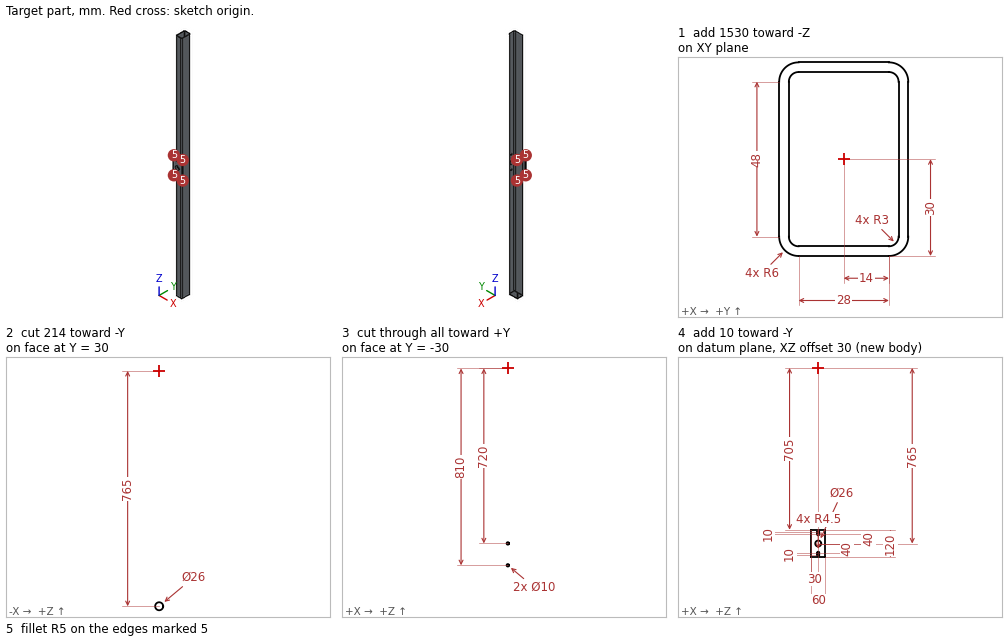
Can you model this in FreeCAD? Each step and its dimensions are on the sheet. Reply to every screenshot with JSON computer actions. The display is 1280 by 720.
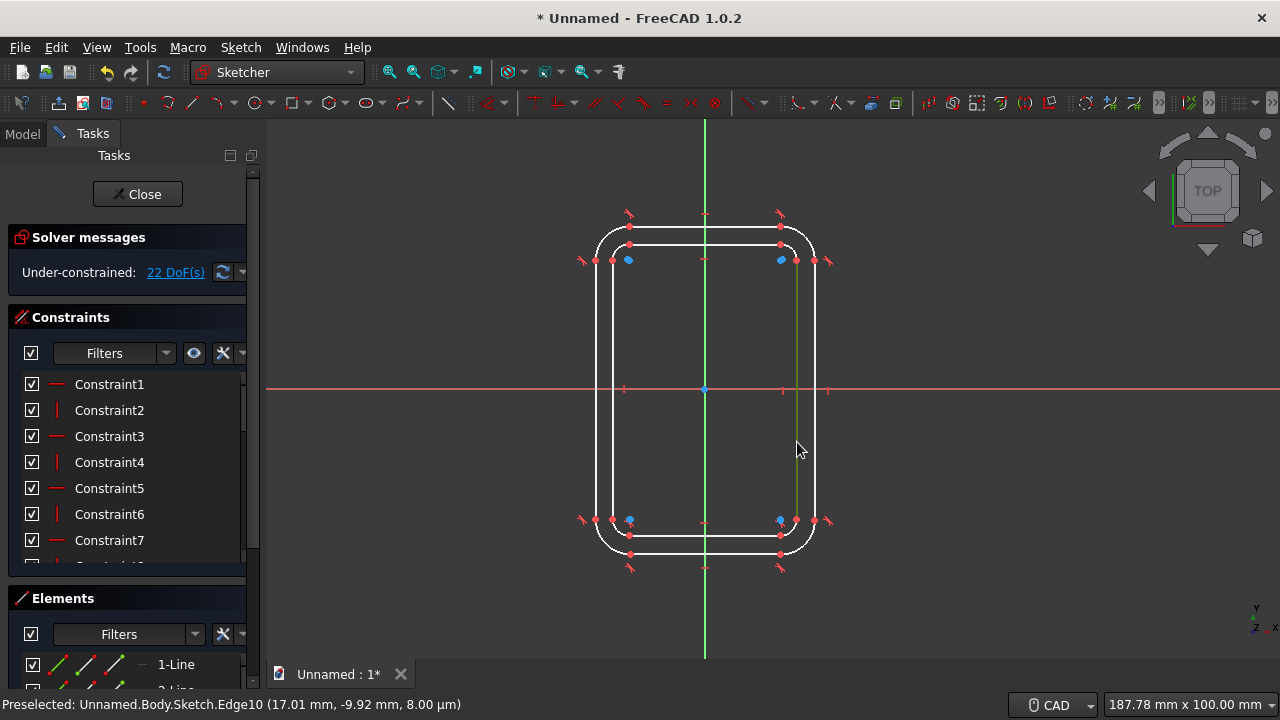
{"action": "left_click", "coordinate": [792, 531]}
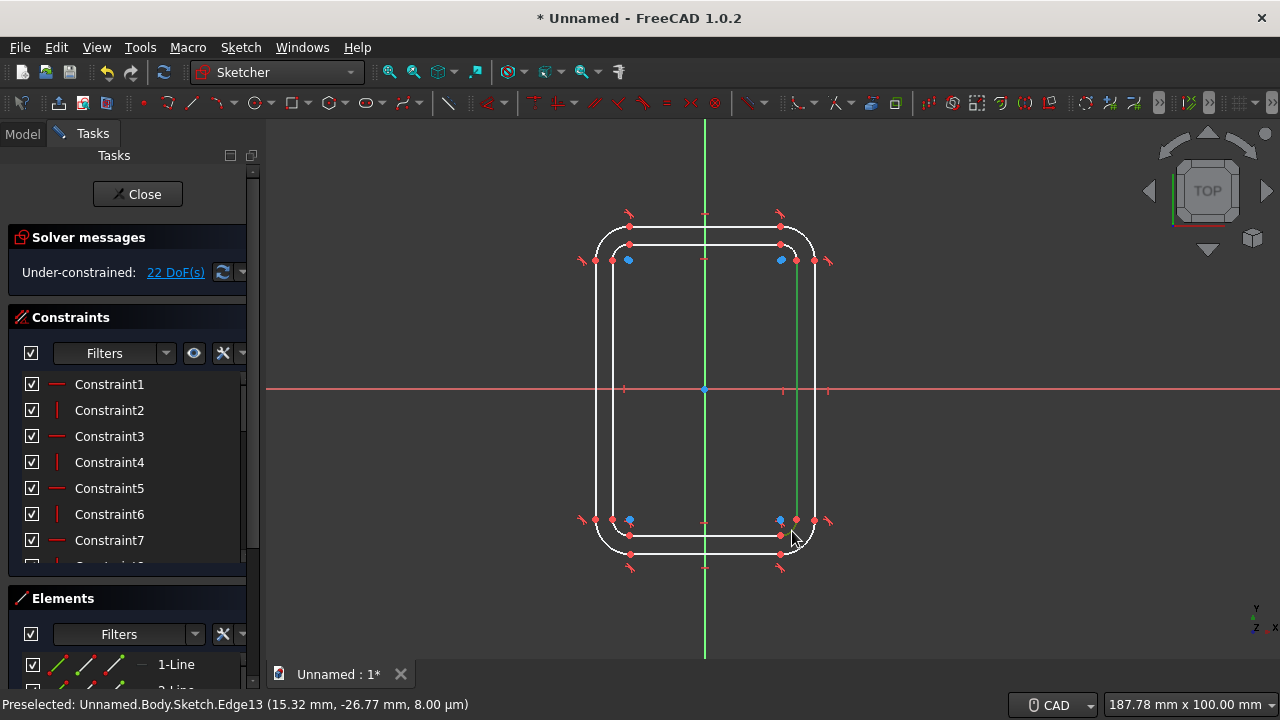
{"action": "left_click", "coordinate": [644, 104]}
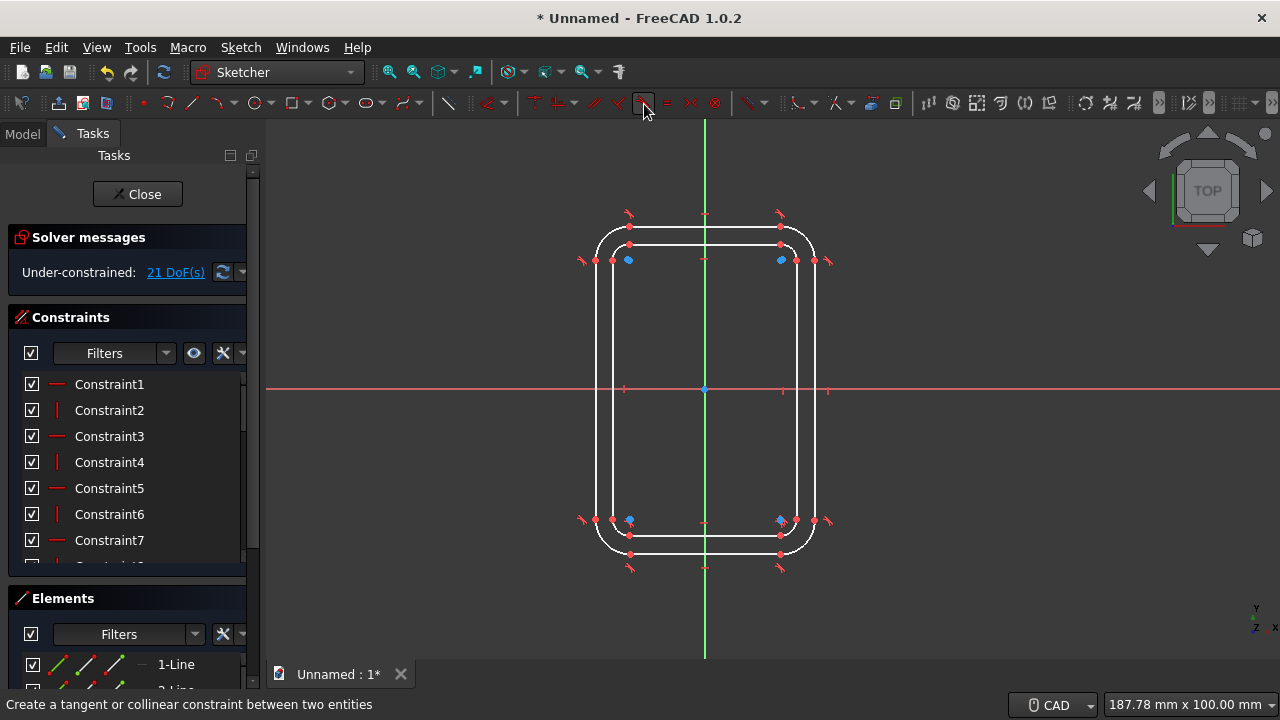
{"action": "left_click", "coordinate": [797, 442]}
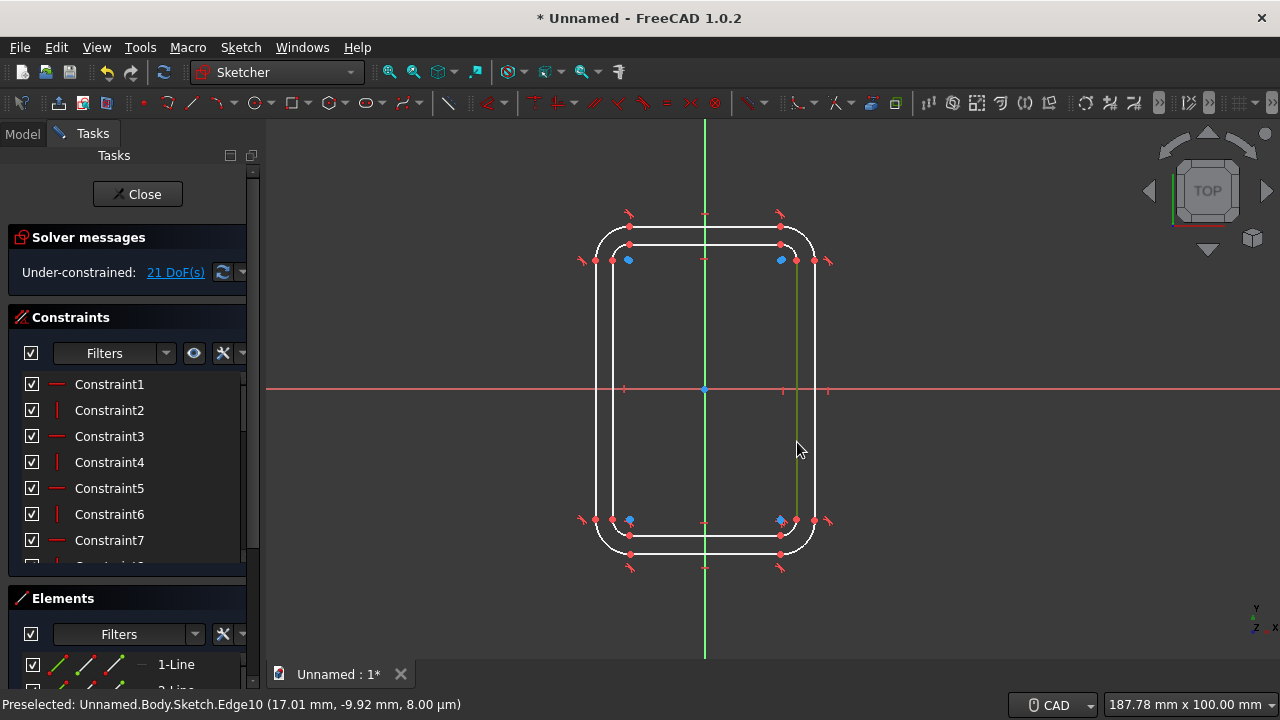
{"action": "left_click", "coordinate": [792, 249]}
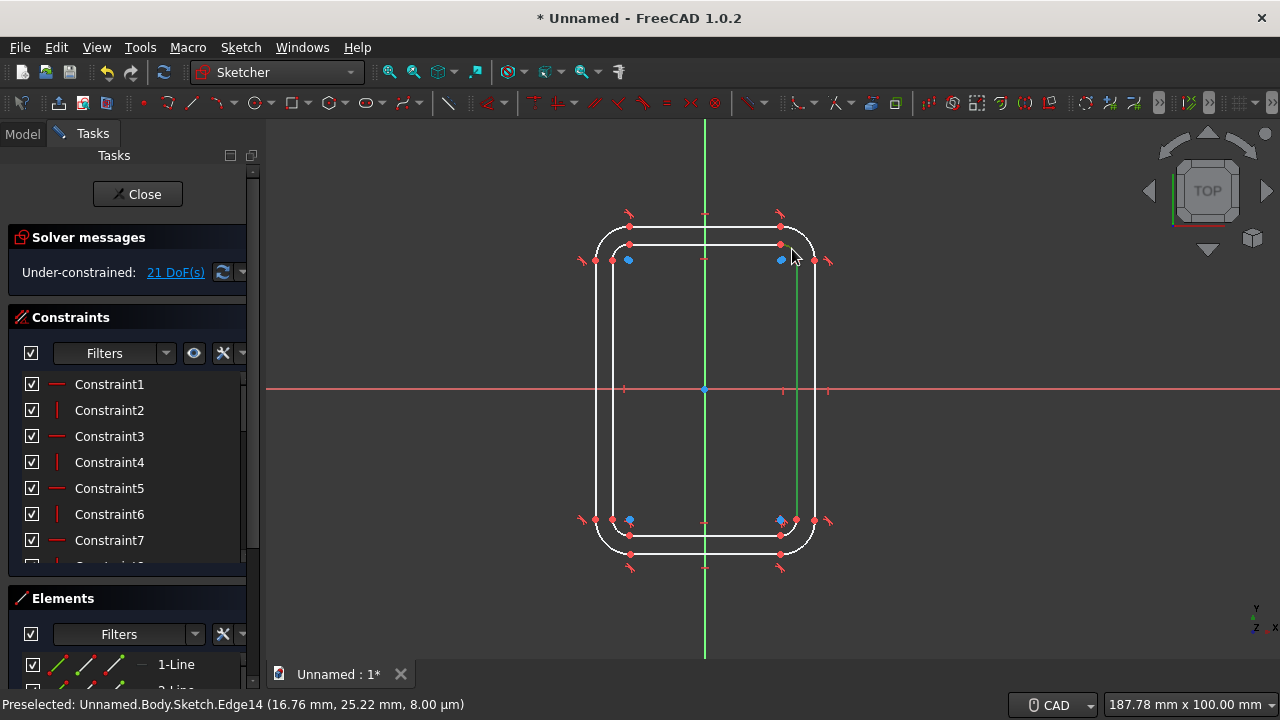
{"action": "left_click", "coordinate": [644, 104]}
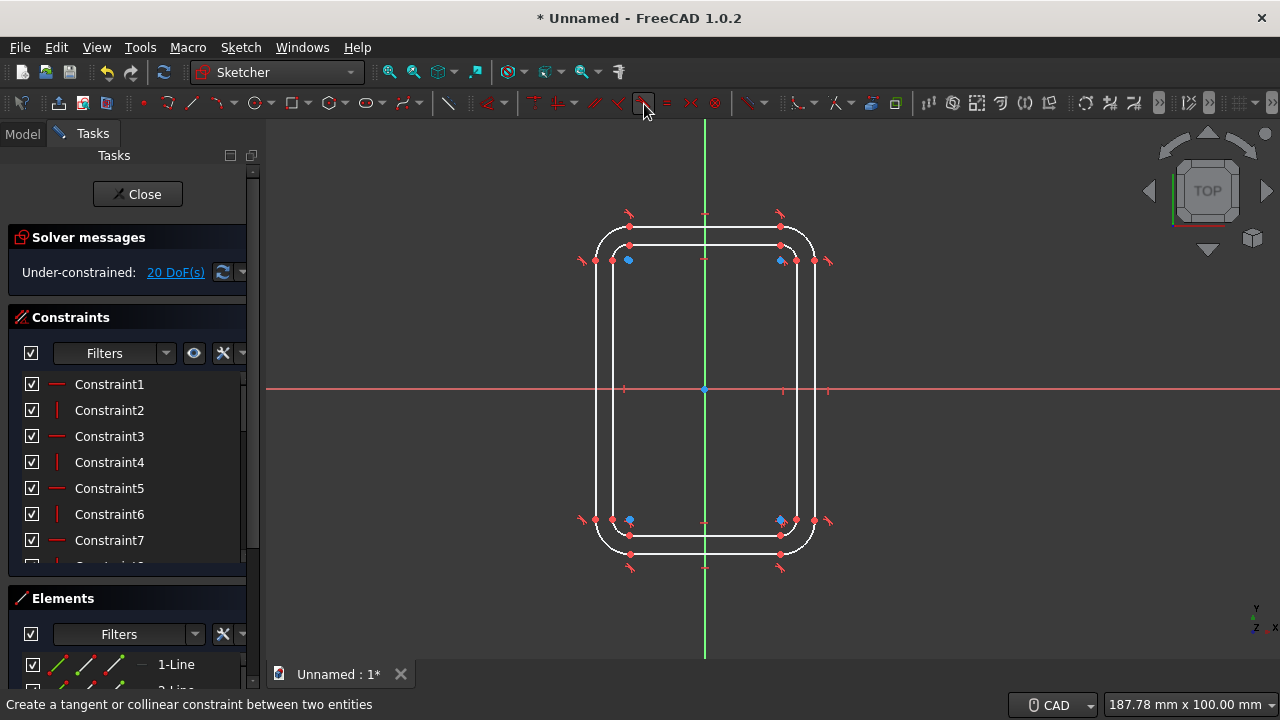
{"action": "left_click", "coordinate": [735, 245]}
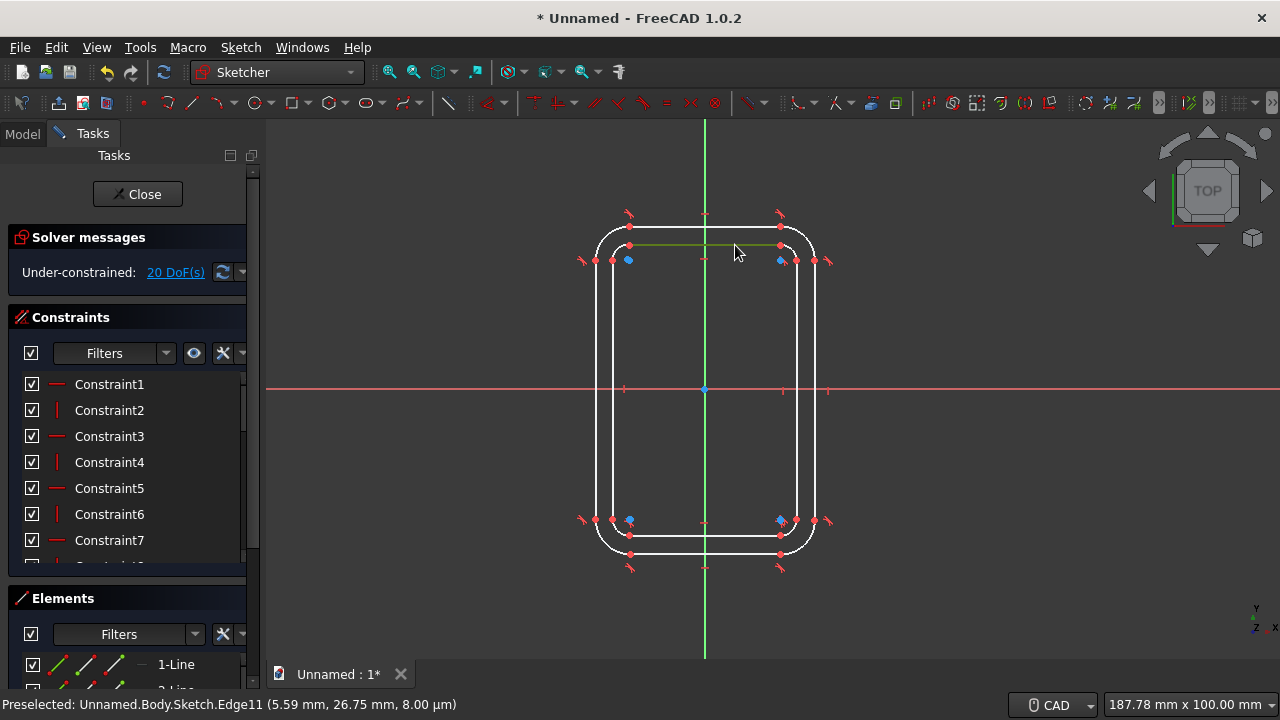
{"action": "left_click", "coordinate": [792, 249]}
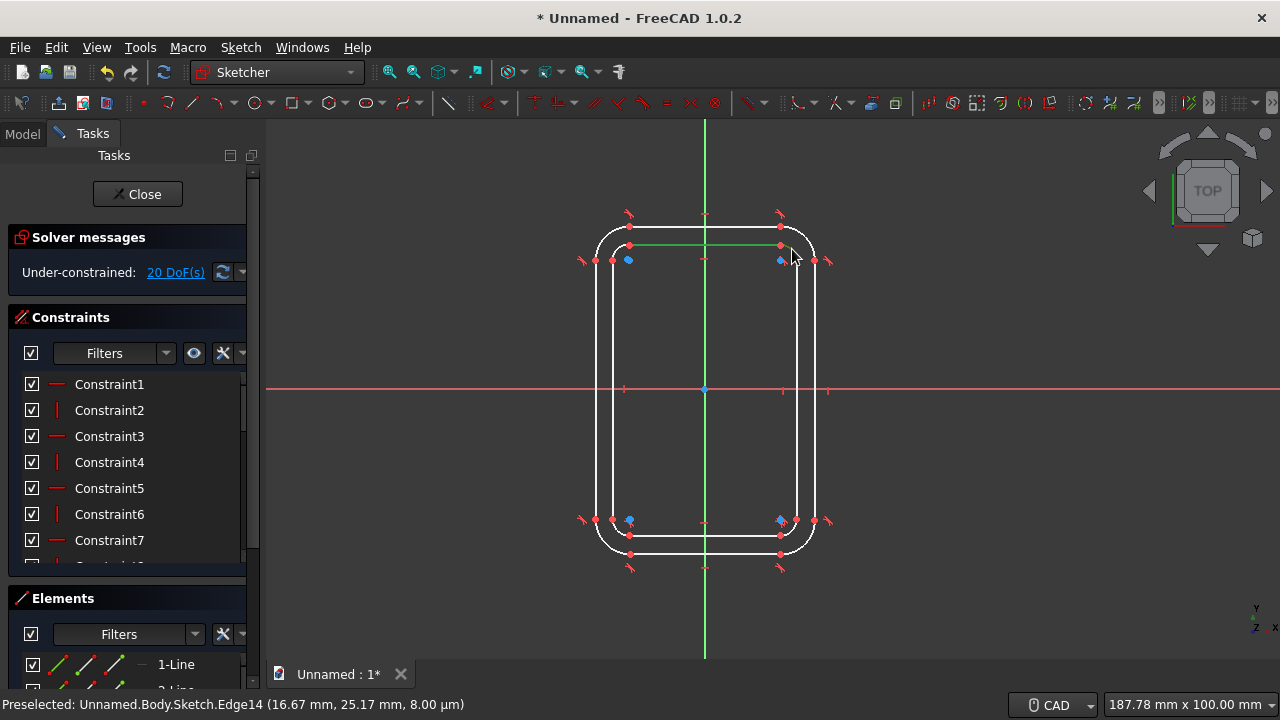
{"action": "left_click", "coordinate": [644, 104]}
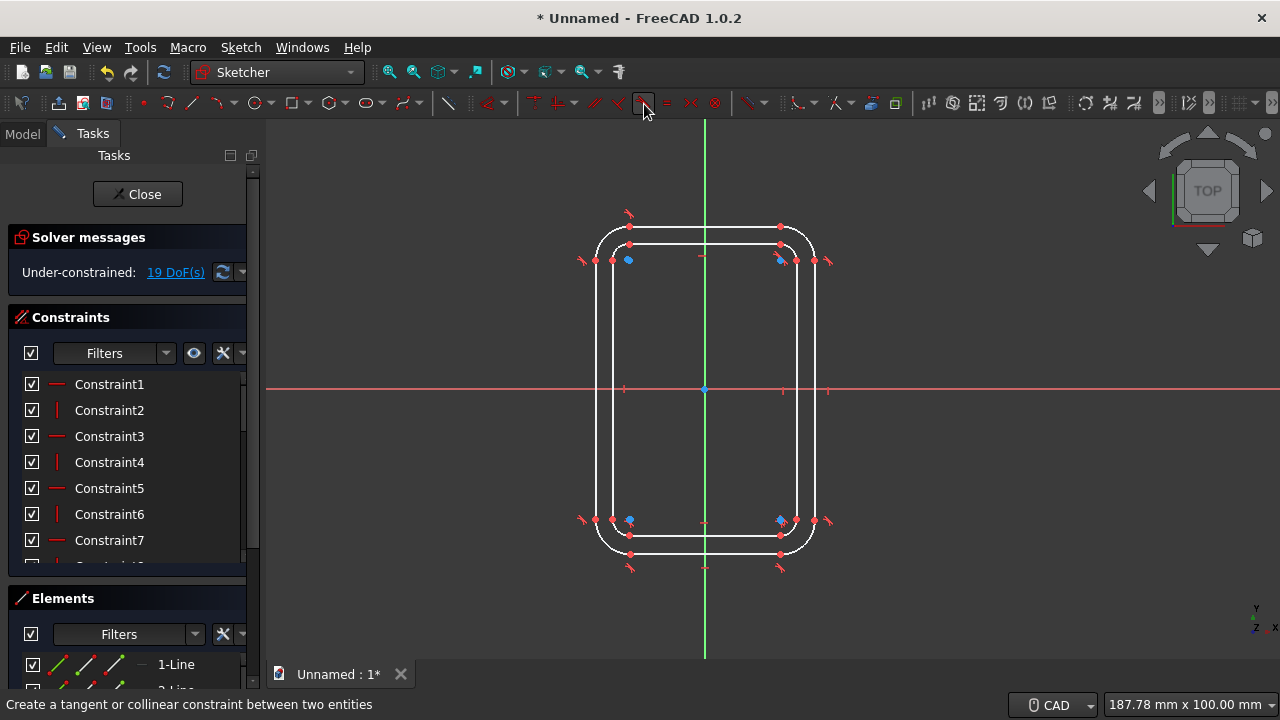
{"action": "left_click", "coordinate": [735, 244]}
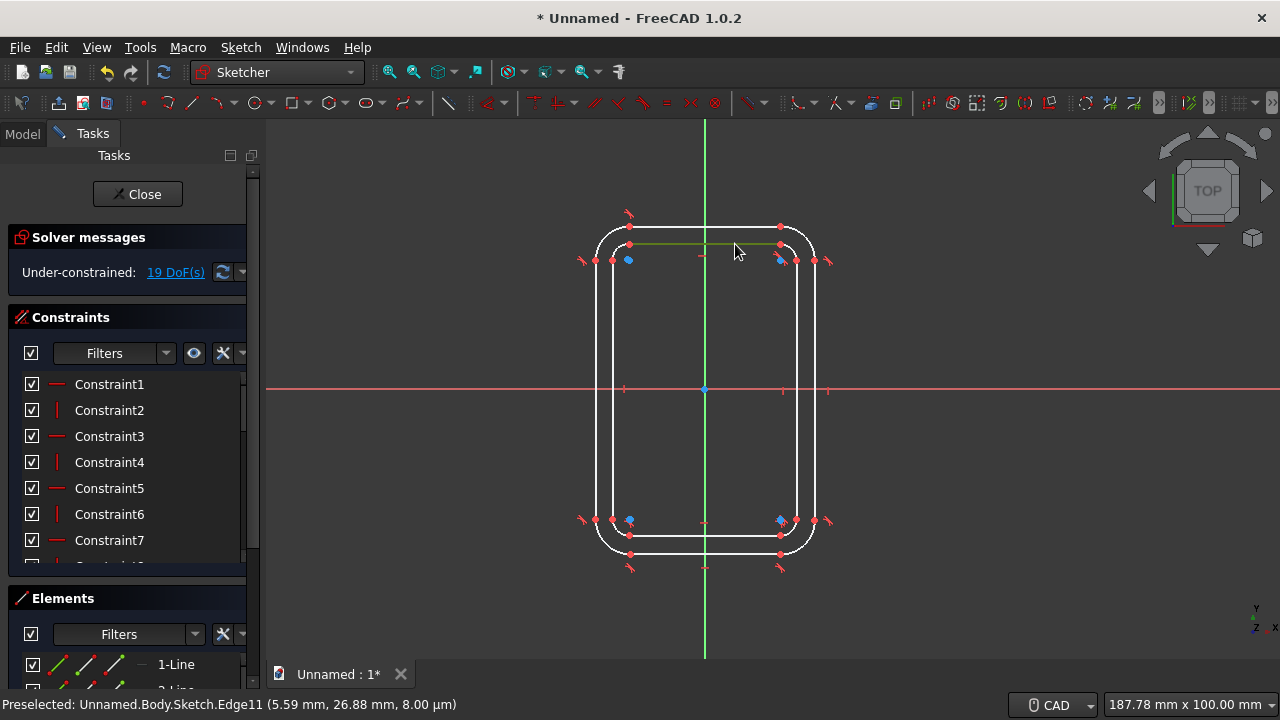
{"action": "left_click", "coordinate": [617, 249]}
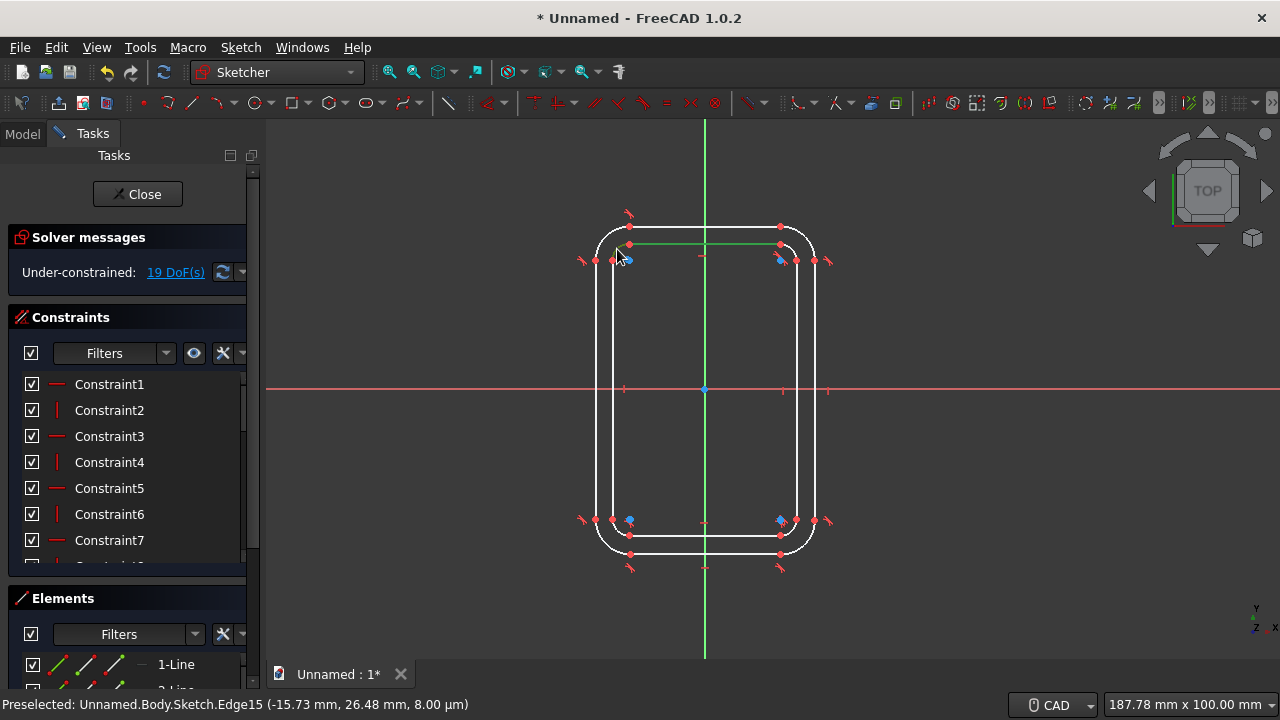
{"action": "left_click", "coordinate": [644, 104]}